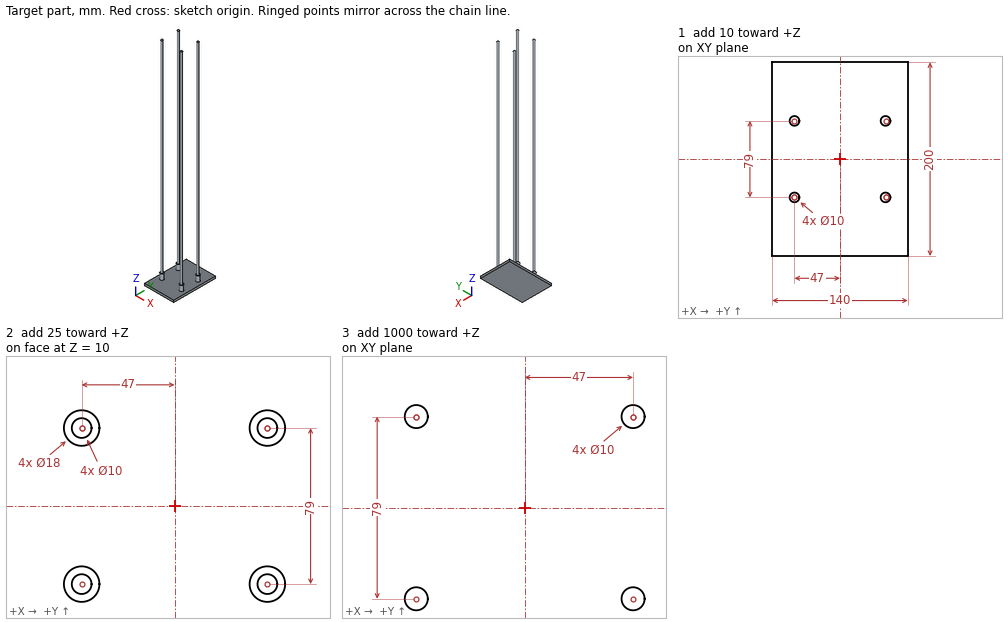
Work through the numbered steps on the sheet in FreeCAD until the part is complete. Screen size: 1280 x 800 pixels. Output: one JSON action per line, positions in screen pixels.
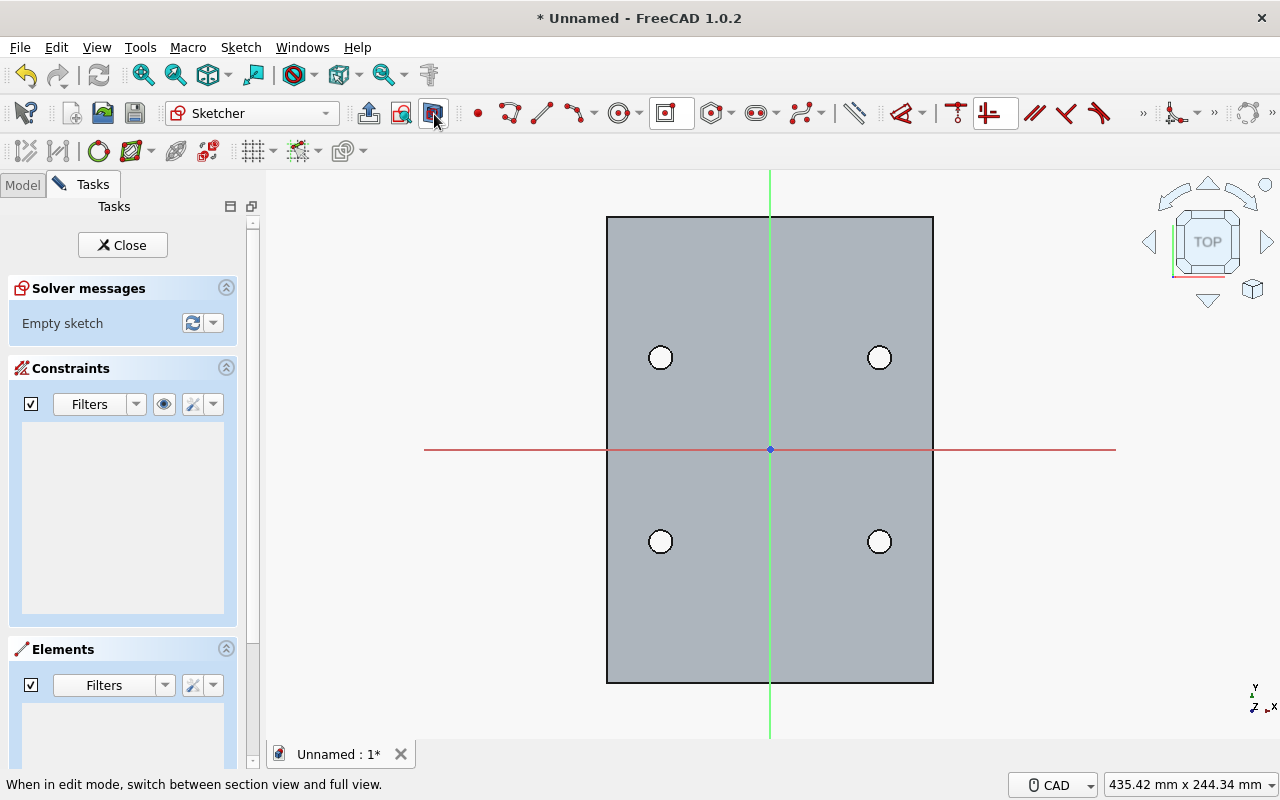
{"action": "scroll", "coordinate": [850, 444], "scroll_direction": "up", "scroll_amount": 3}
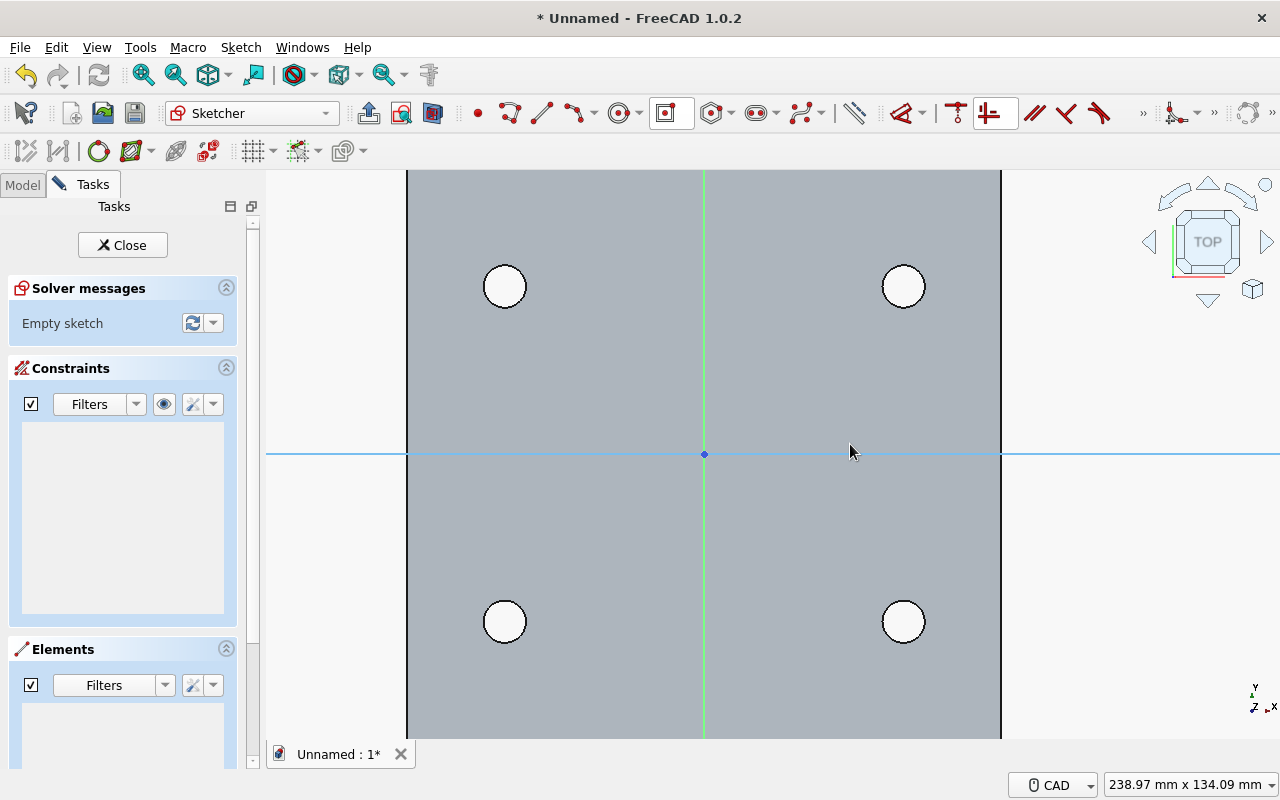
{"action": "left_click", "coordinate": [620, 114]}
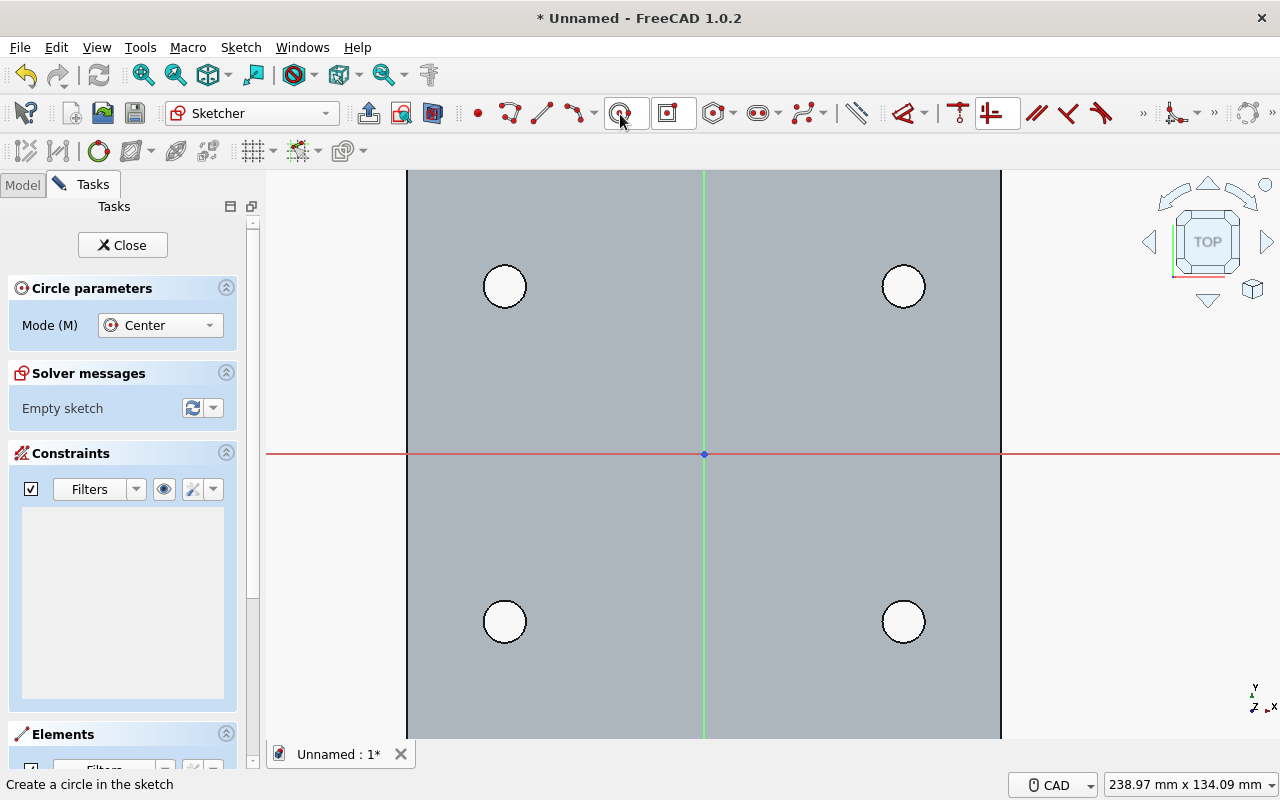
{"action": "left_click", "coordinate": [904, 286]}
{"action": "left_click", "coordinate": [919, 271]}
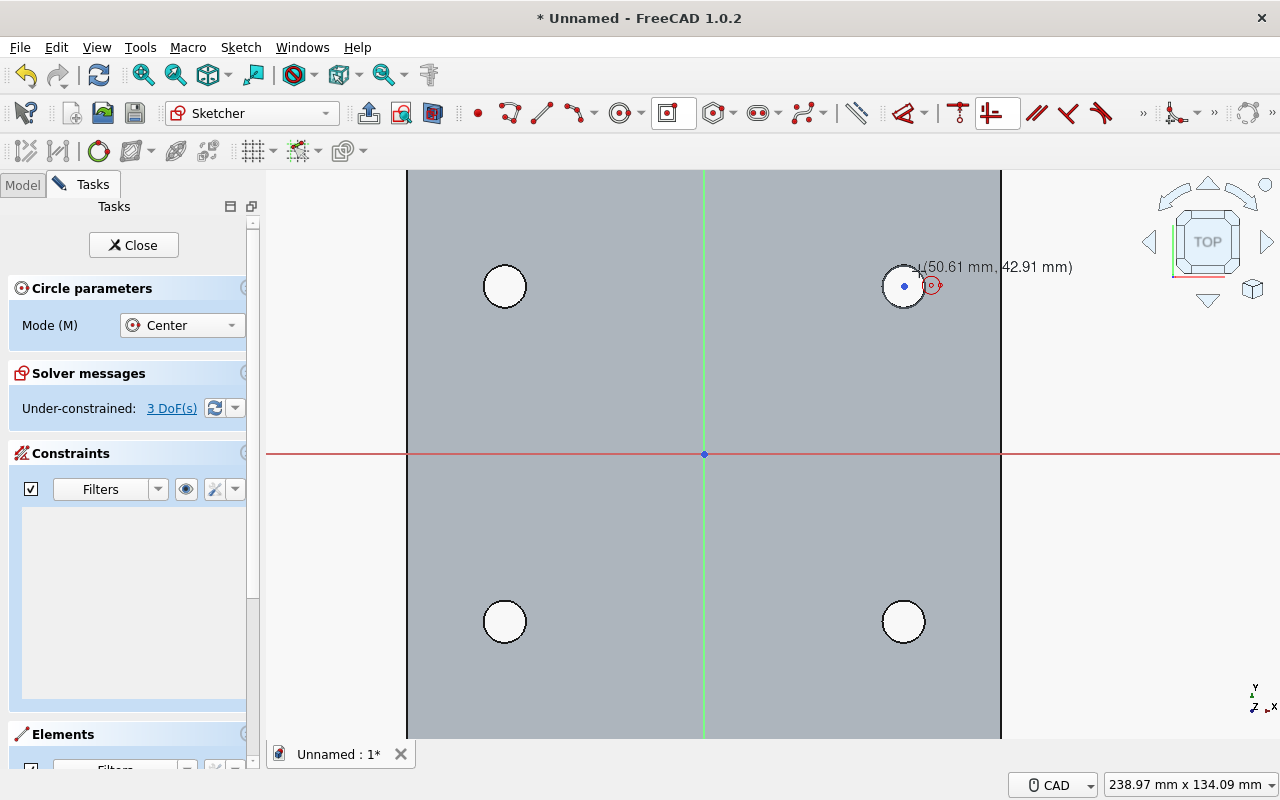
{"action": "left_click", "coordinate": [505, 286]}
{"action": "left_click", "coordinate": [520, 271]}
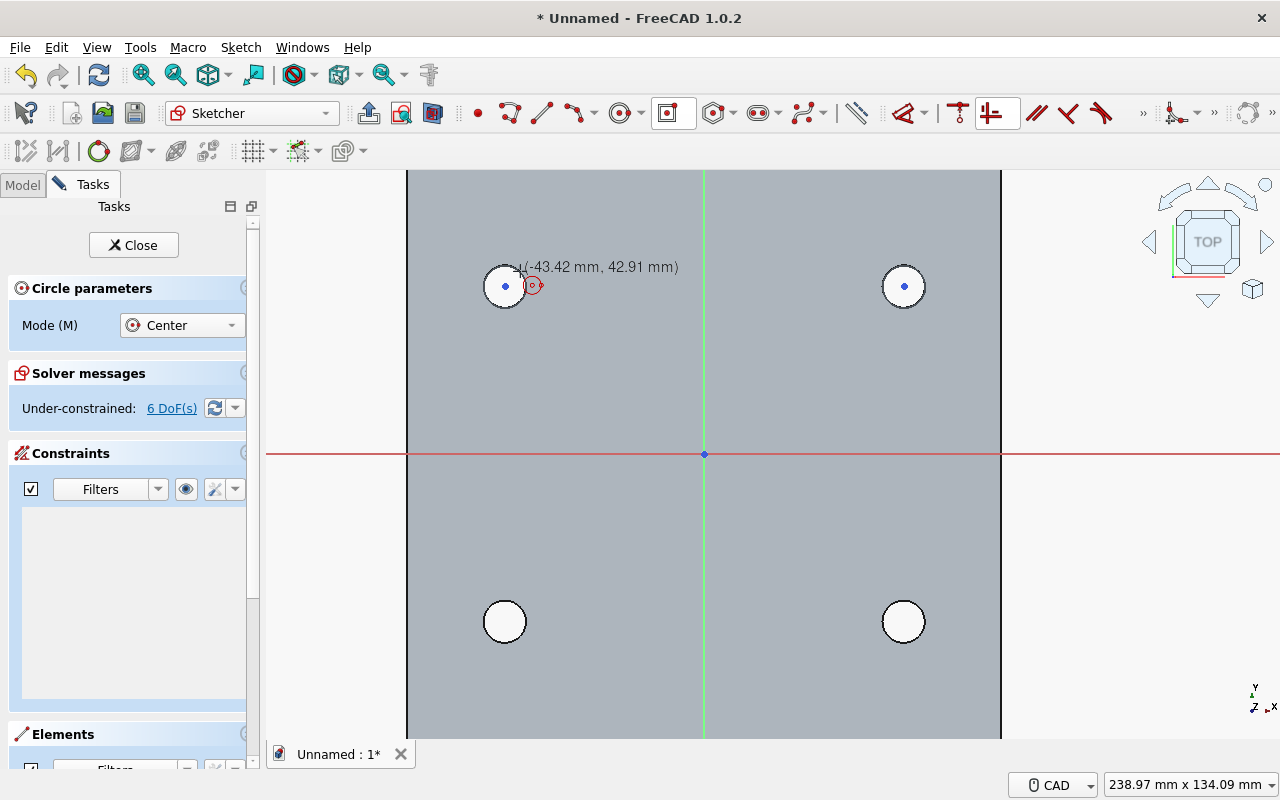
{"action": "left_click", "coordinate": [505, 622]}
{"action": "left_click", "coordinate": [520, 607]}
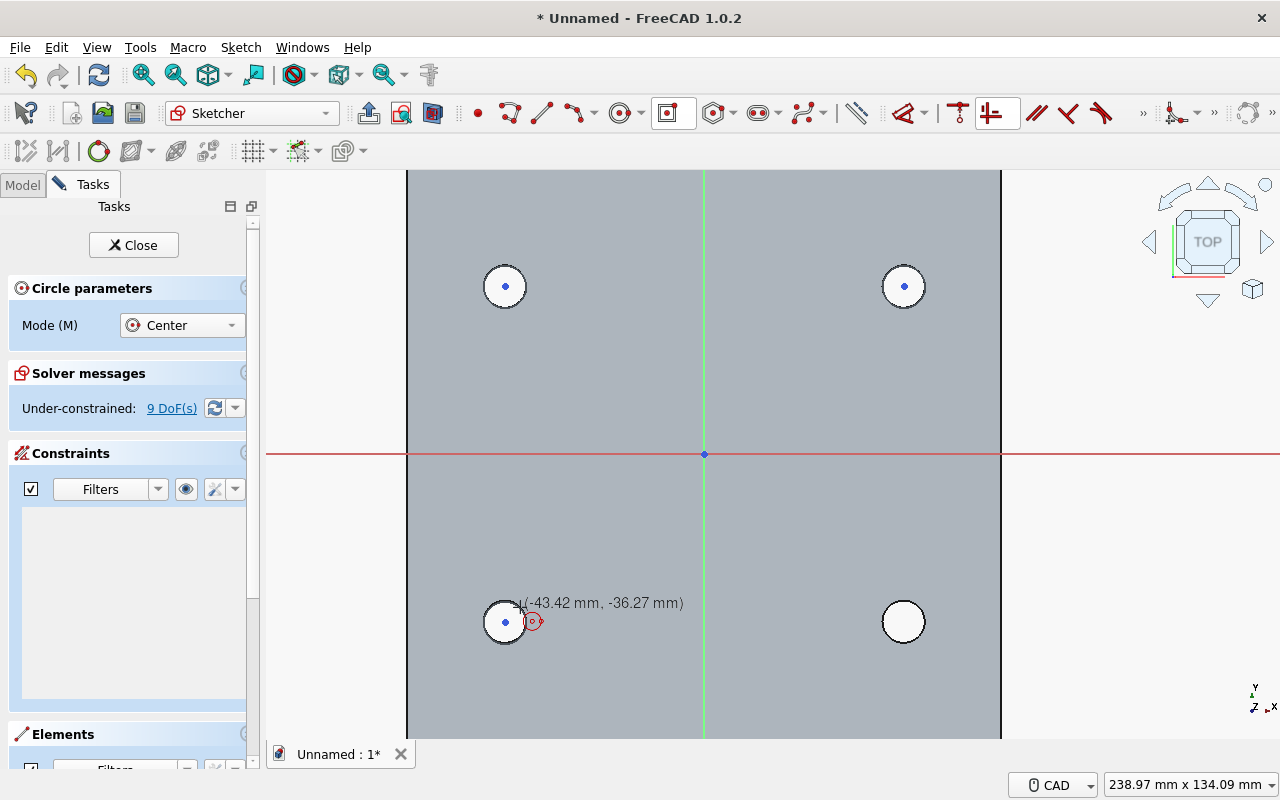
{"action": "left_click", "coordinate": [904, 622]}
{"action": "left_click", "coordinate": [919, 607]}
{"action": "key", "text": "Escape"}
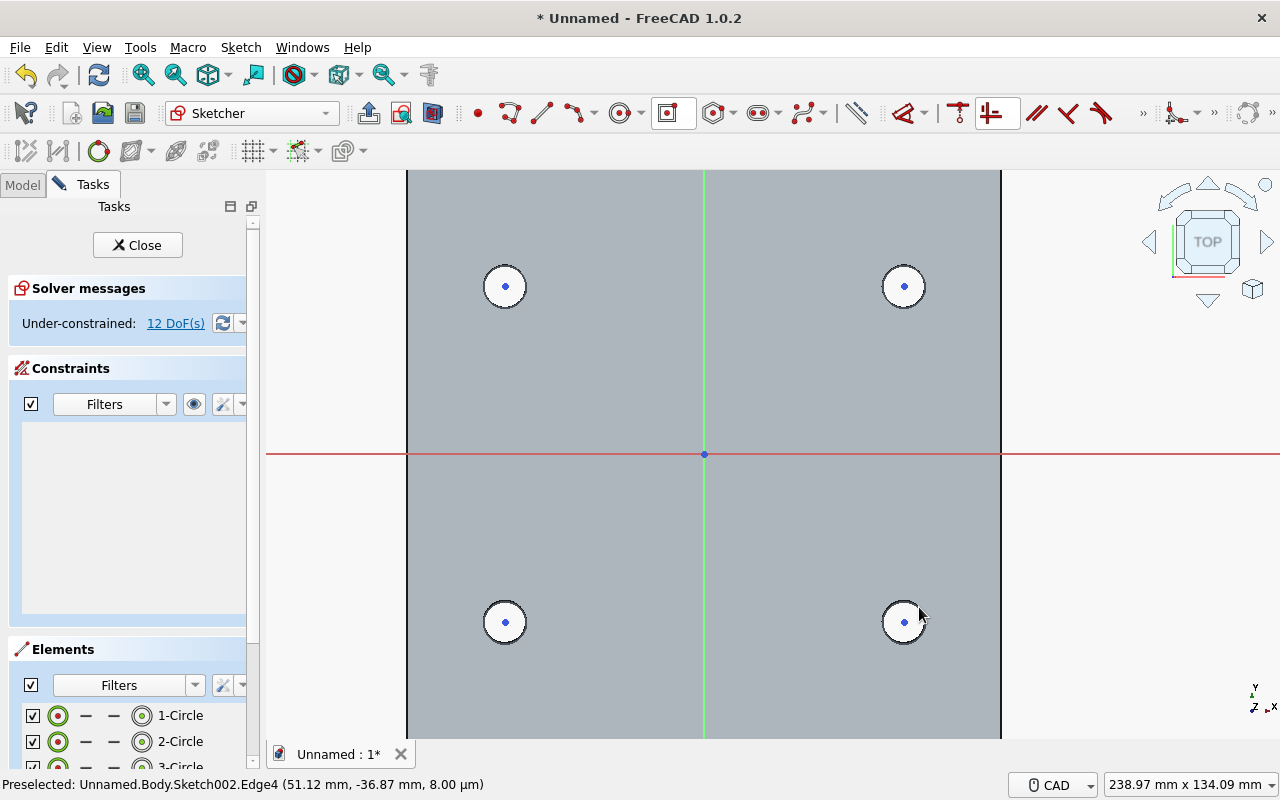
{"action": "left_click", "coordinate": [919, 272]}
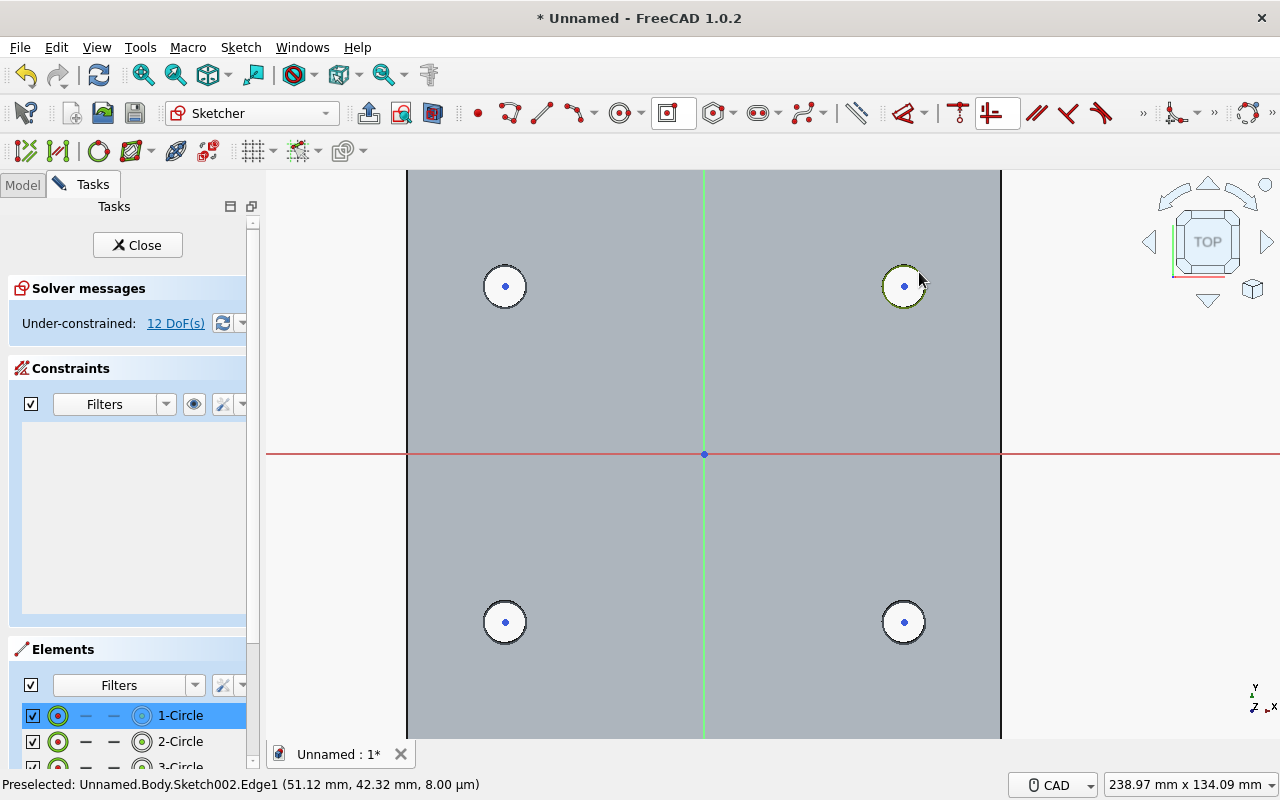
{"action": "left_click", "coordinate": [520, 272]}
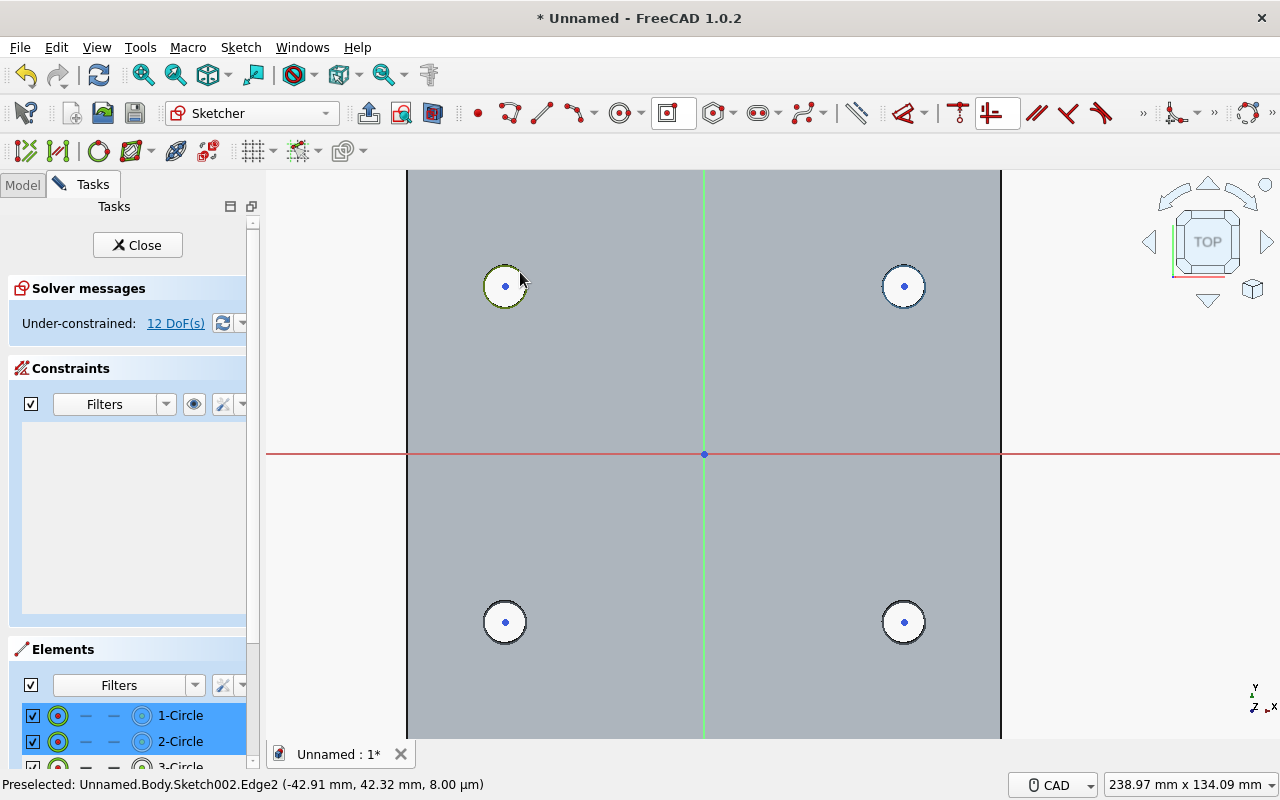
{"action": "left_click", "coordinate": [520, 608]}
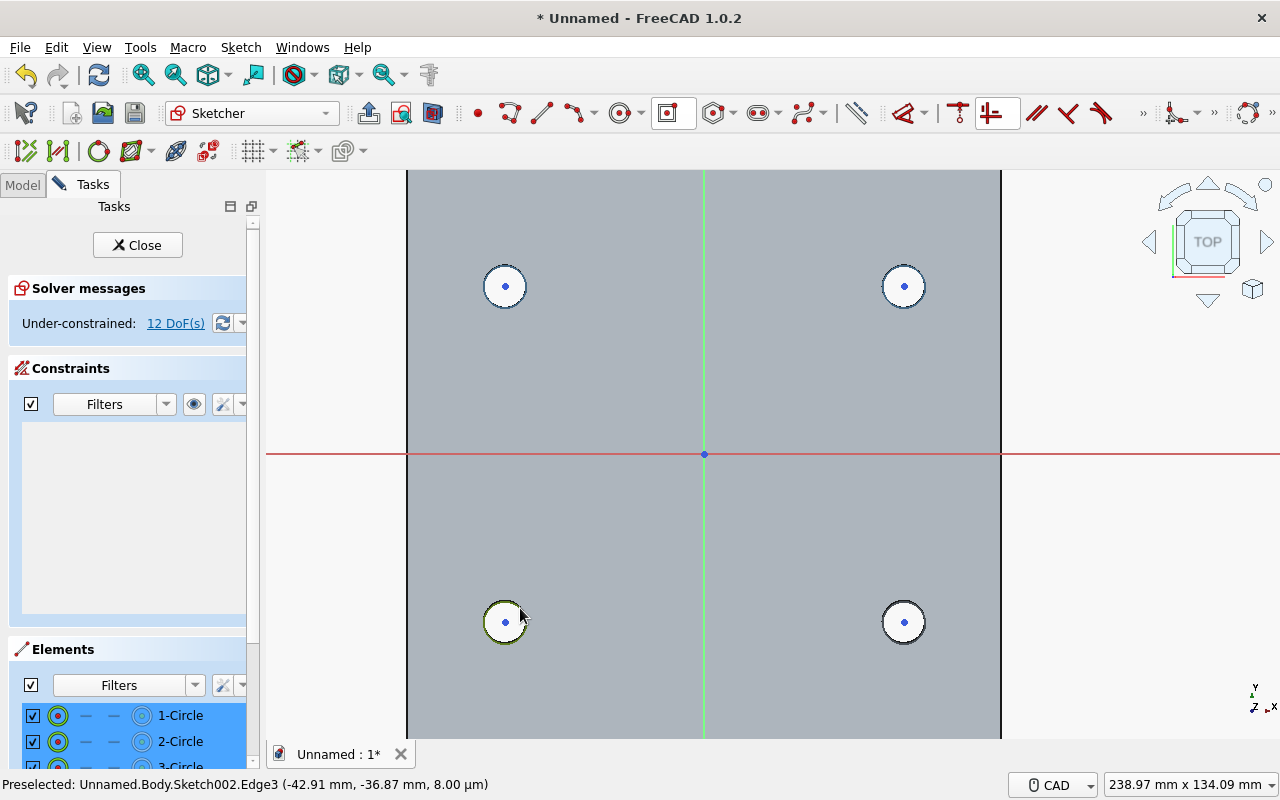
{"action": "left_click", "coordinate": [919, 608]}